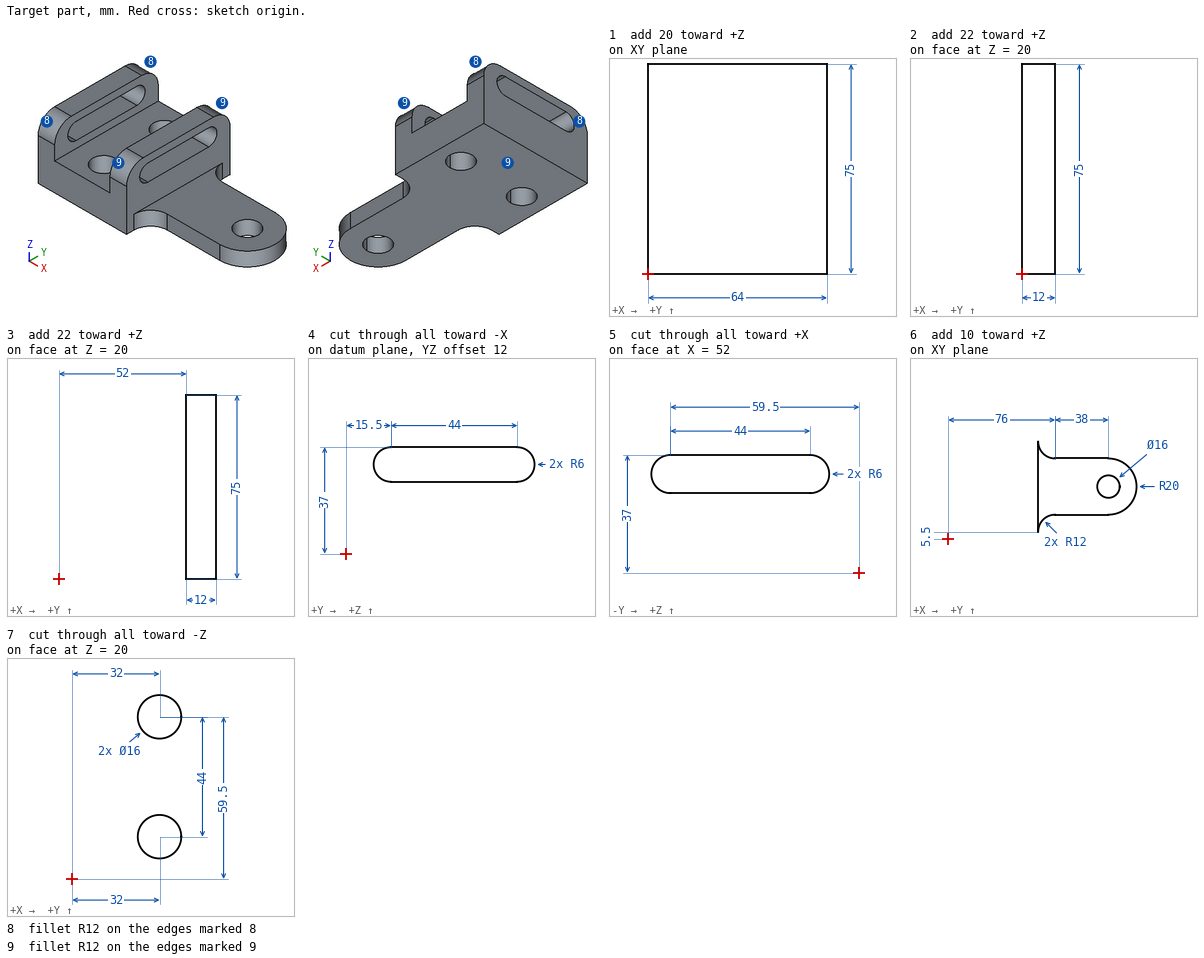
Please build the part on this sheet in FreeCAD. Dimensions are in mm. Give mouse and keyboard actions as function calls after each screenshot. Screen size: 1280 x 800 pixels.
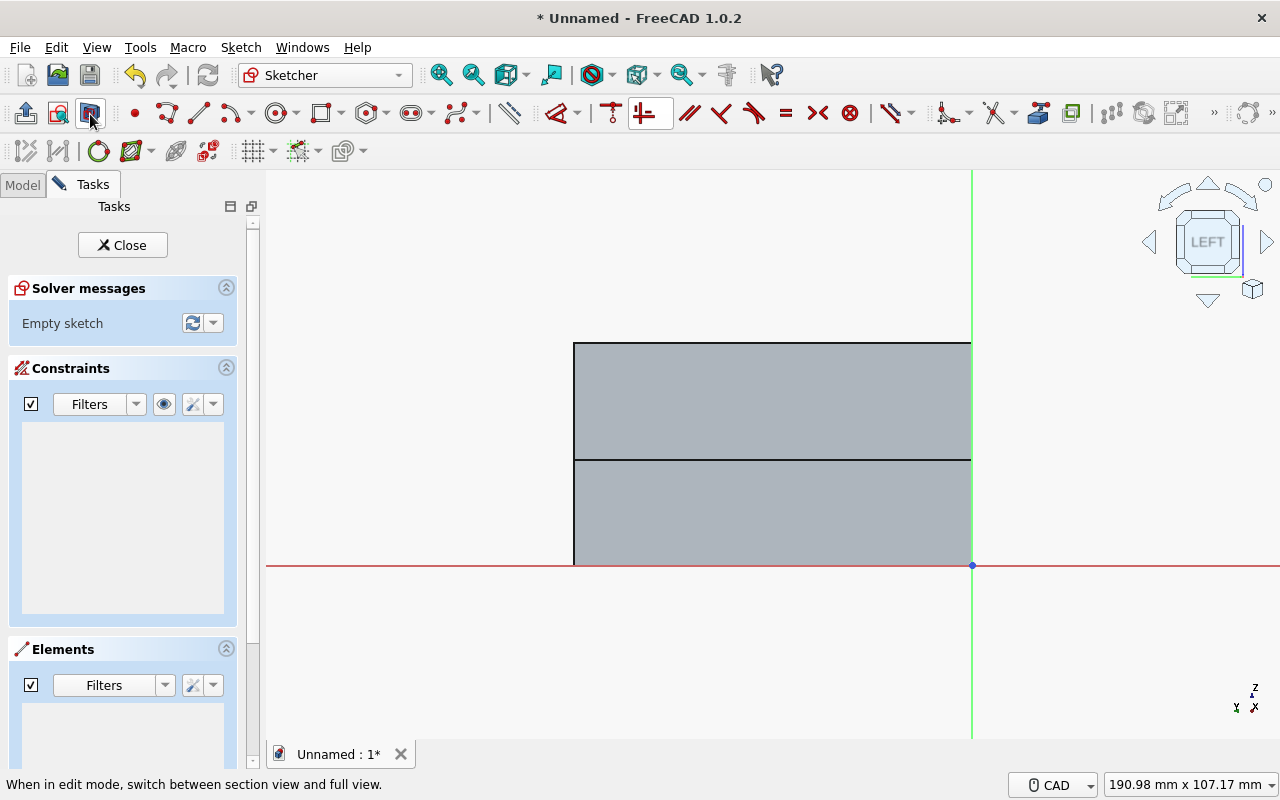
scroll(912, 484, up, 3)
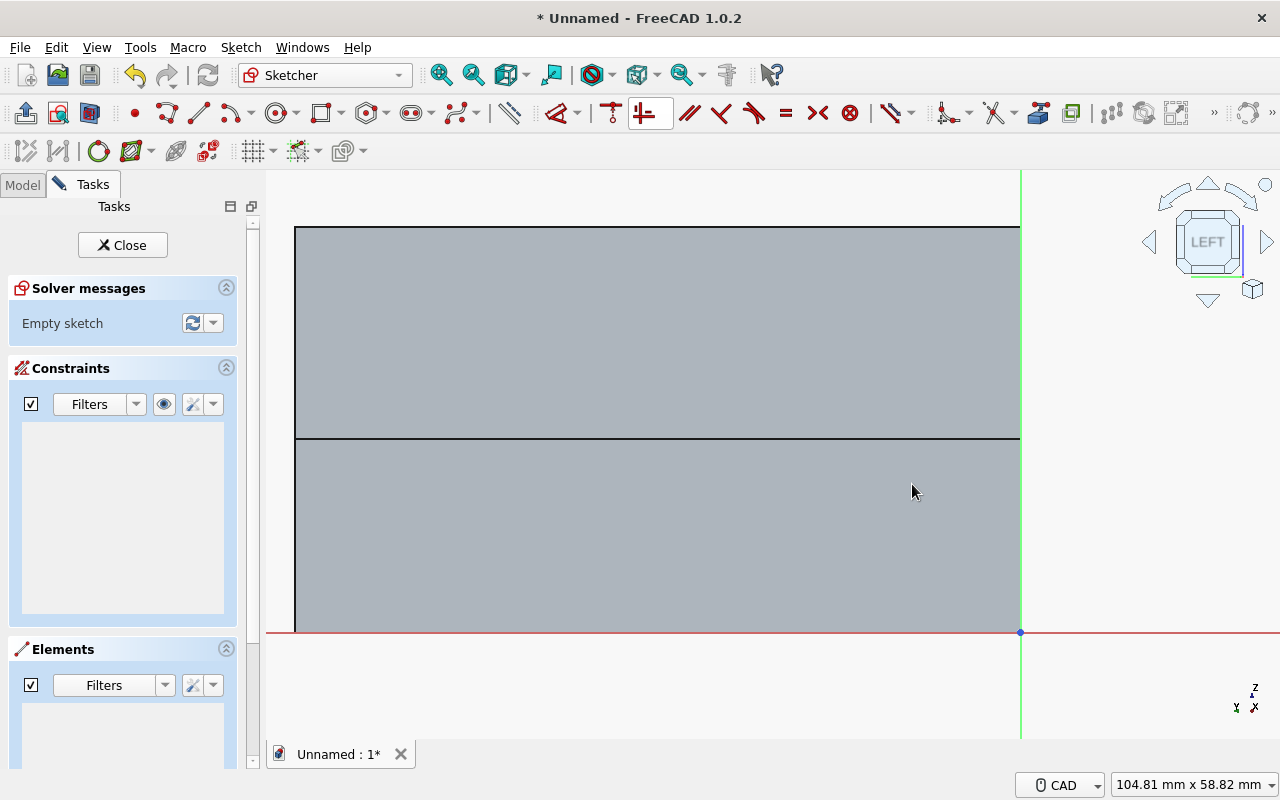
click(412, 114)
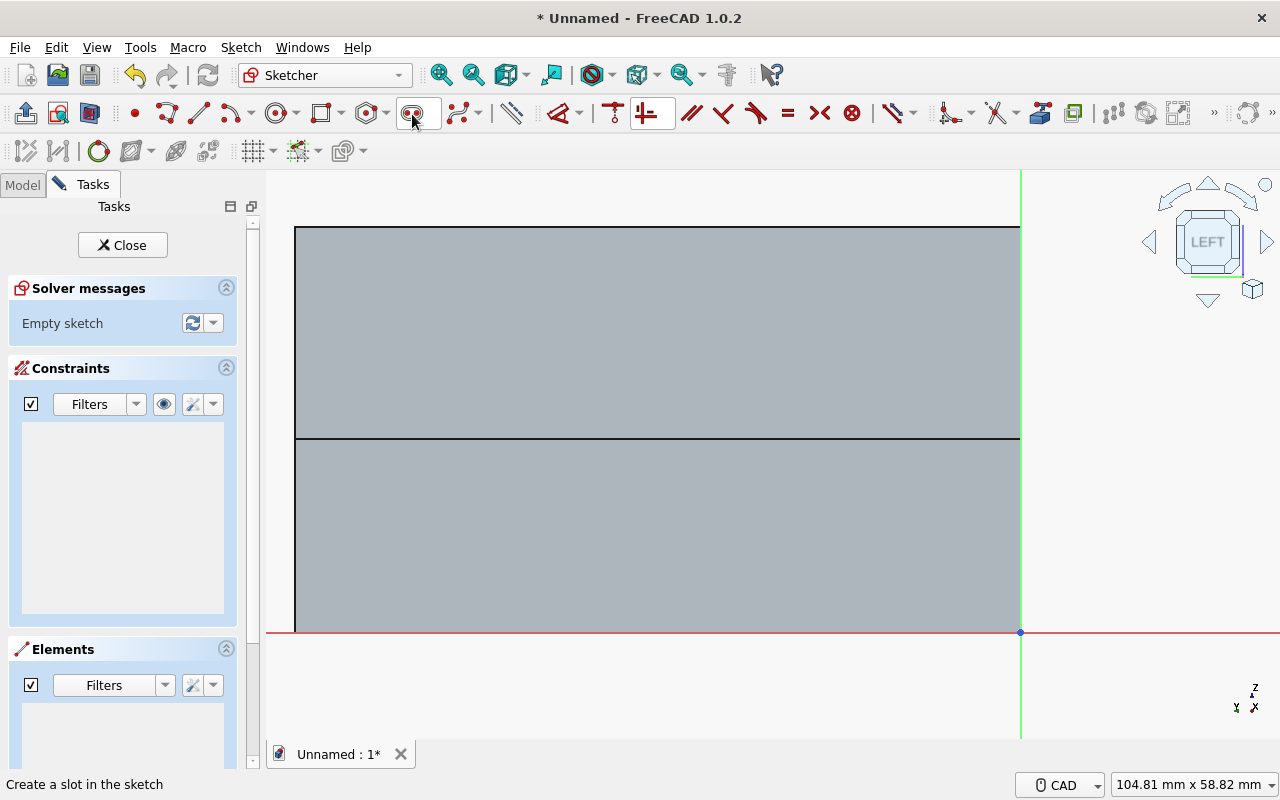
click(445, 333)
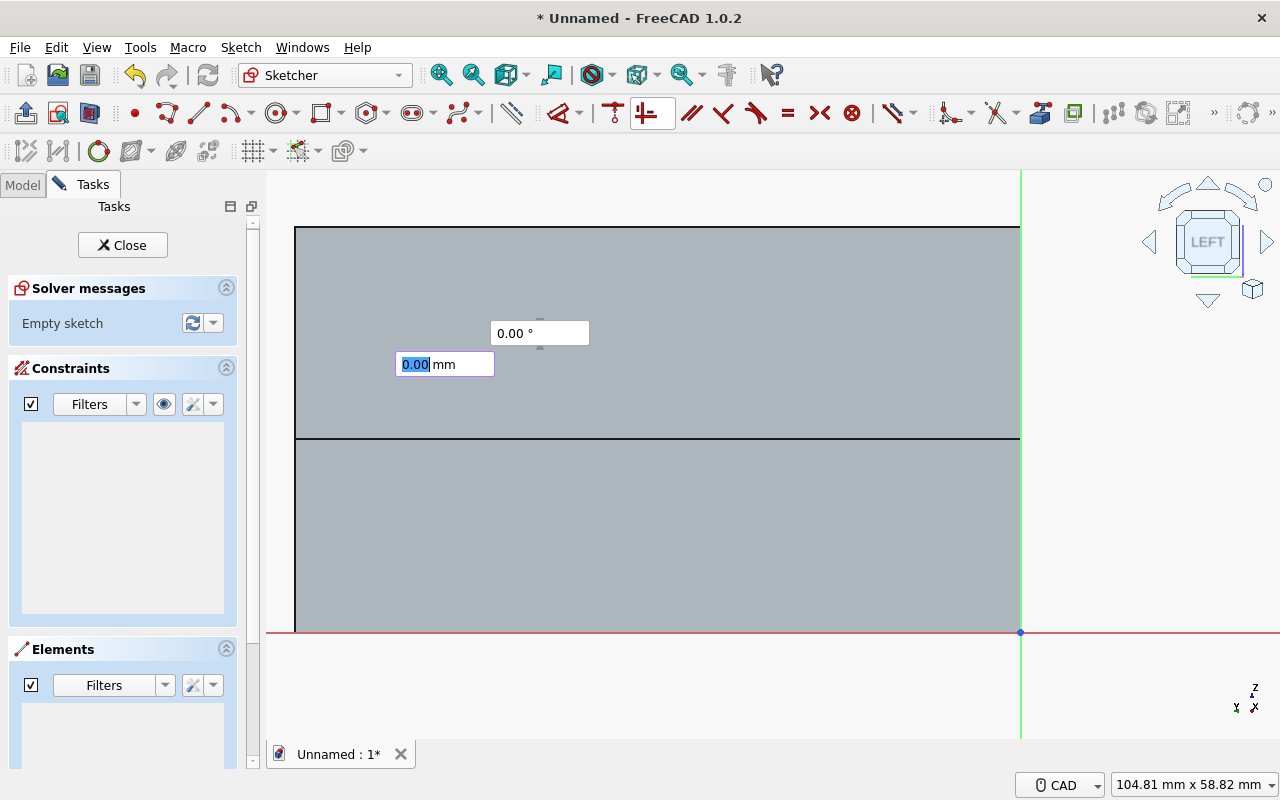
click(871, 333)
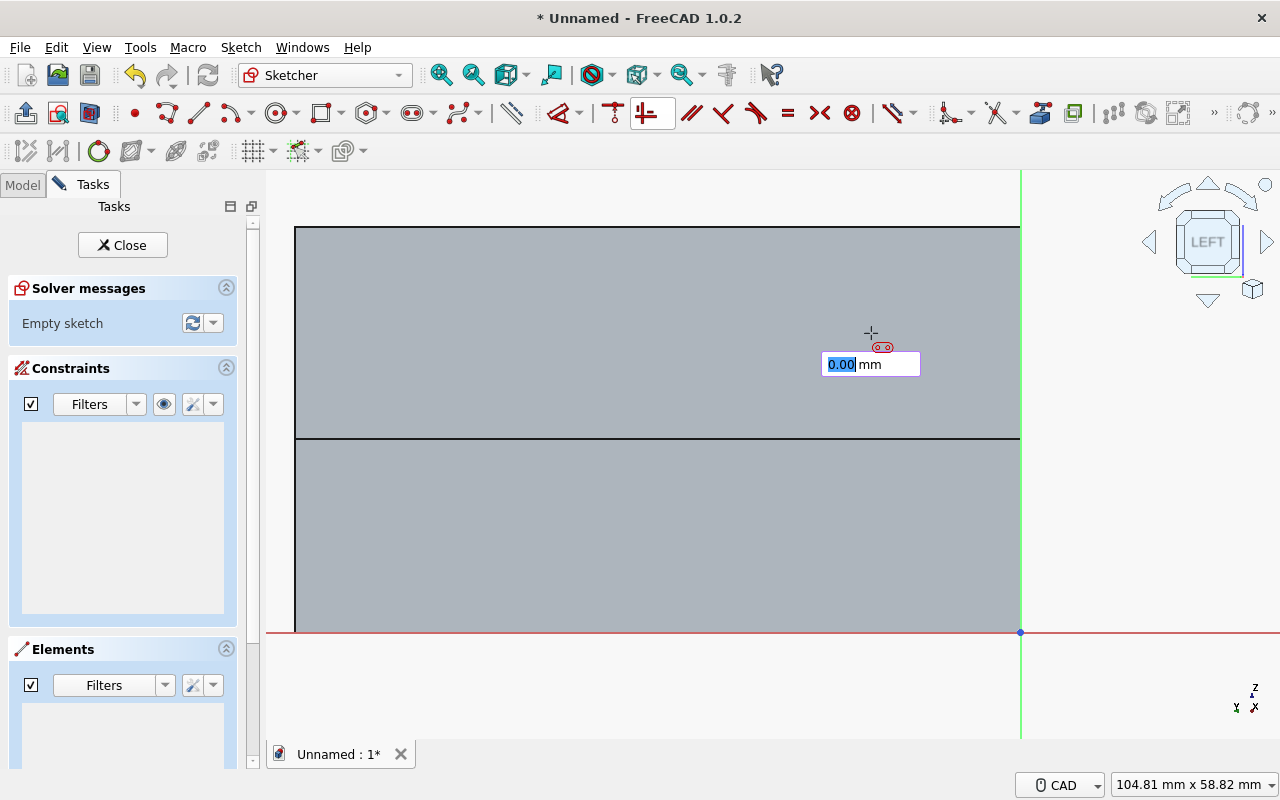
click(658, 391)
key(Escape)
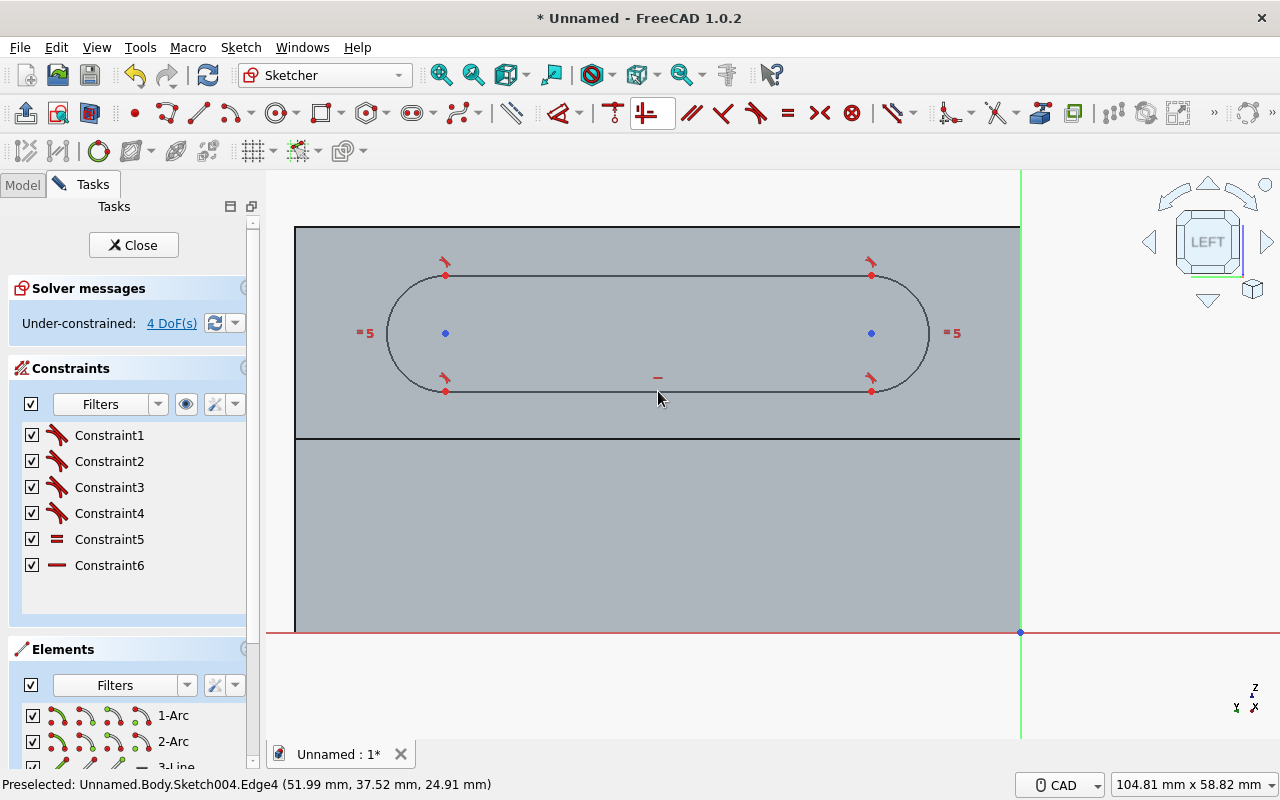
click(558, 114)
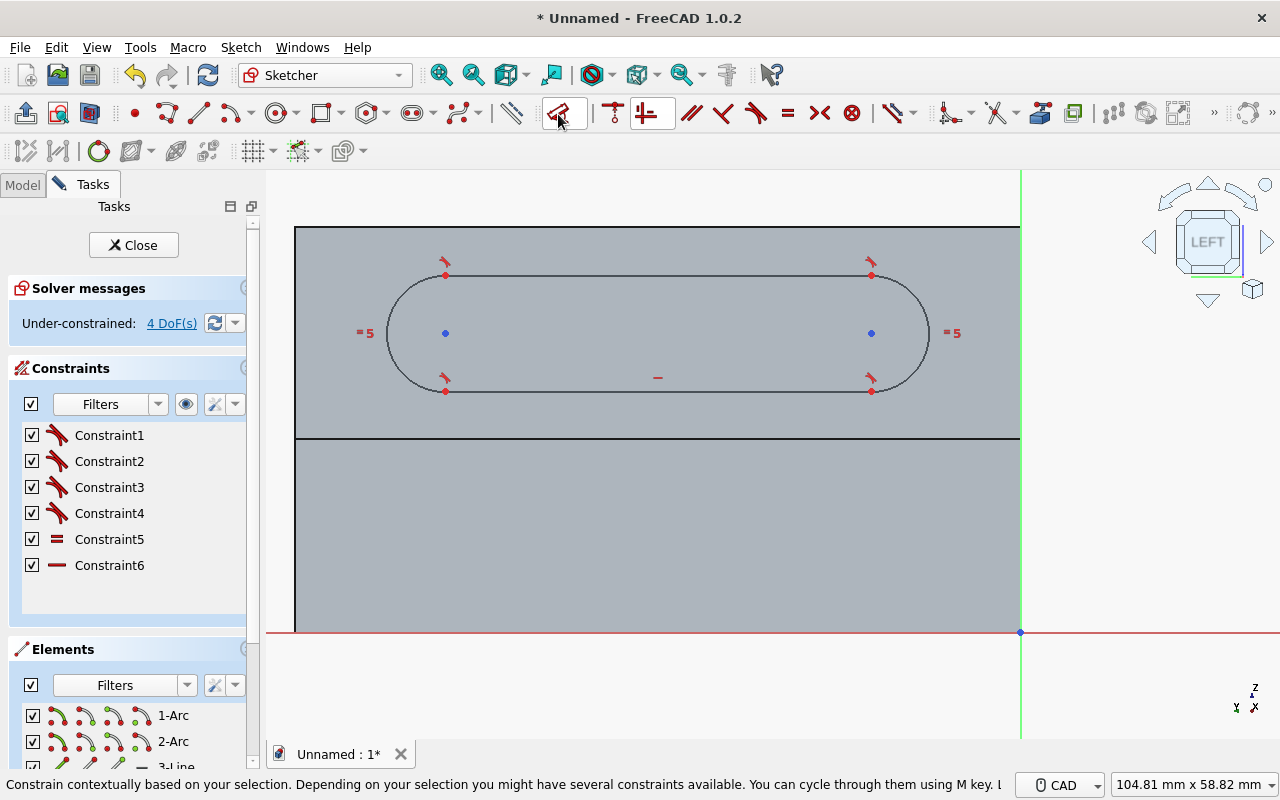
click(398, 300)
click(372, 281)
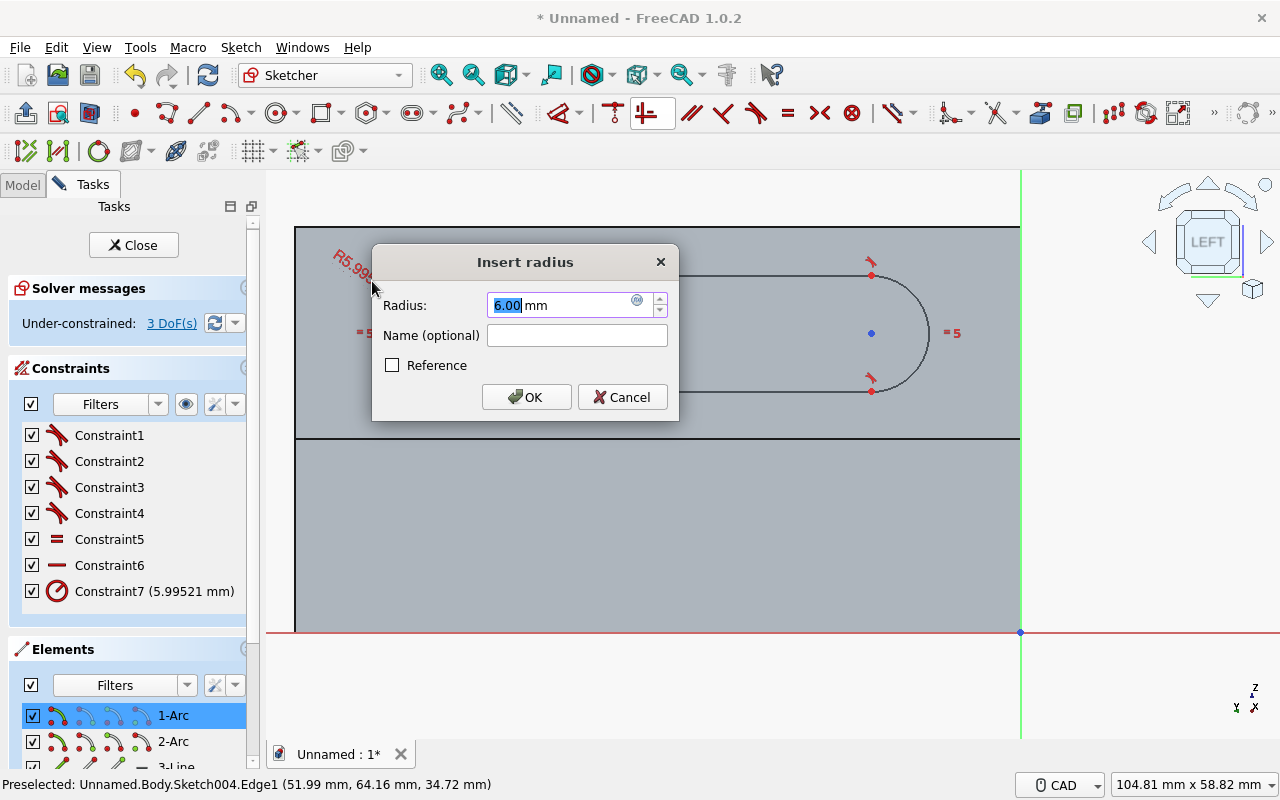
text(6)
key(Return)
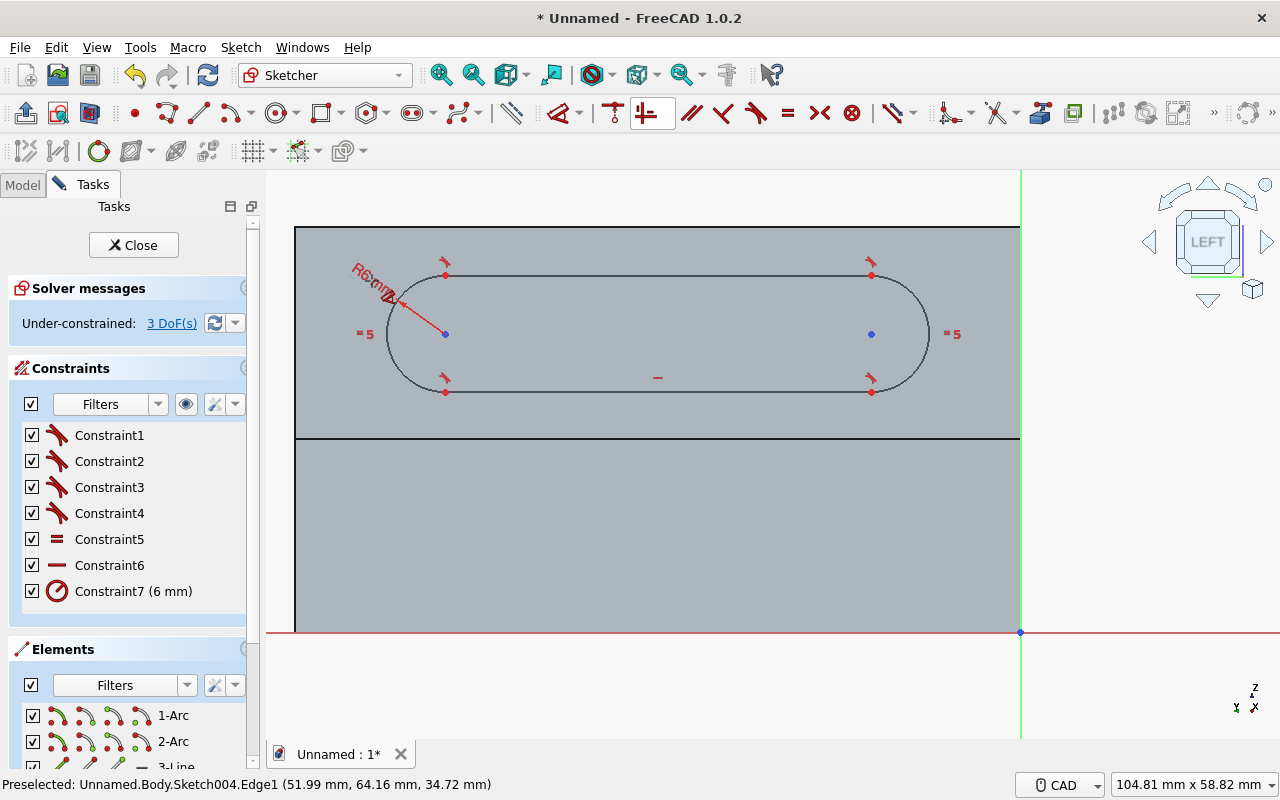
click(573, 276)
click(658, 242)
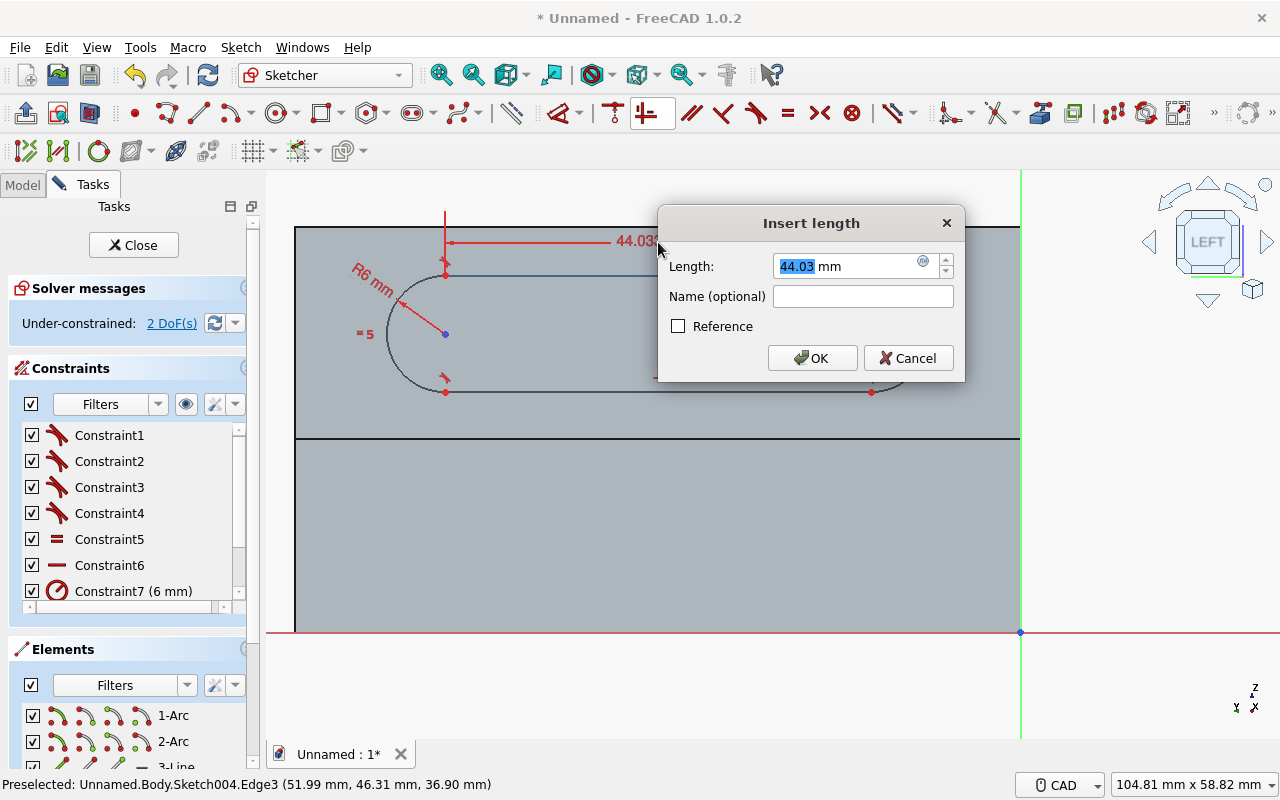
text(44)
key(Return)